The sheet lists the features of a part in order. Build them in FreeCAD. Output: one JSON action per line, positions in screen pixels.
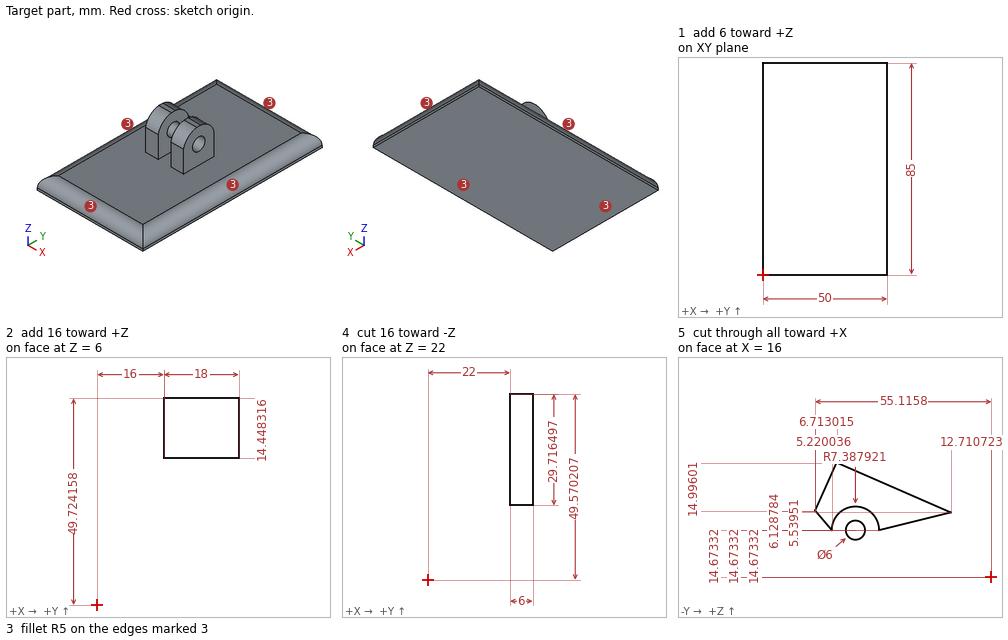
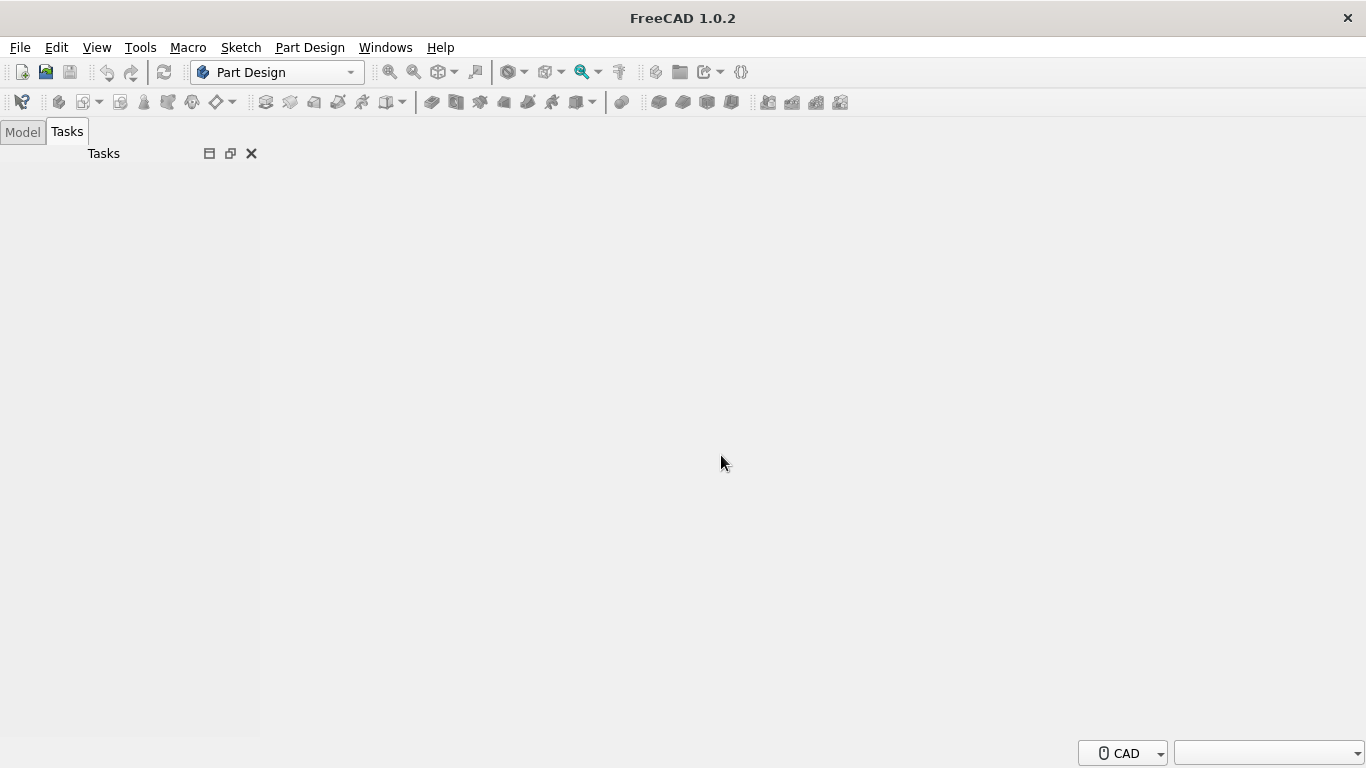
{"action": "key", "text": "ctrl+n"}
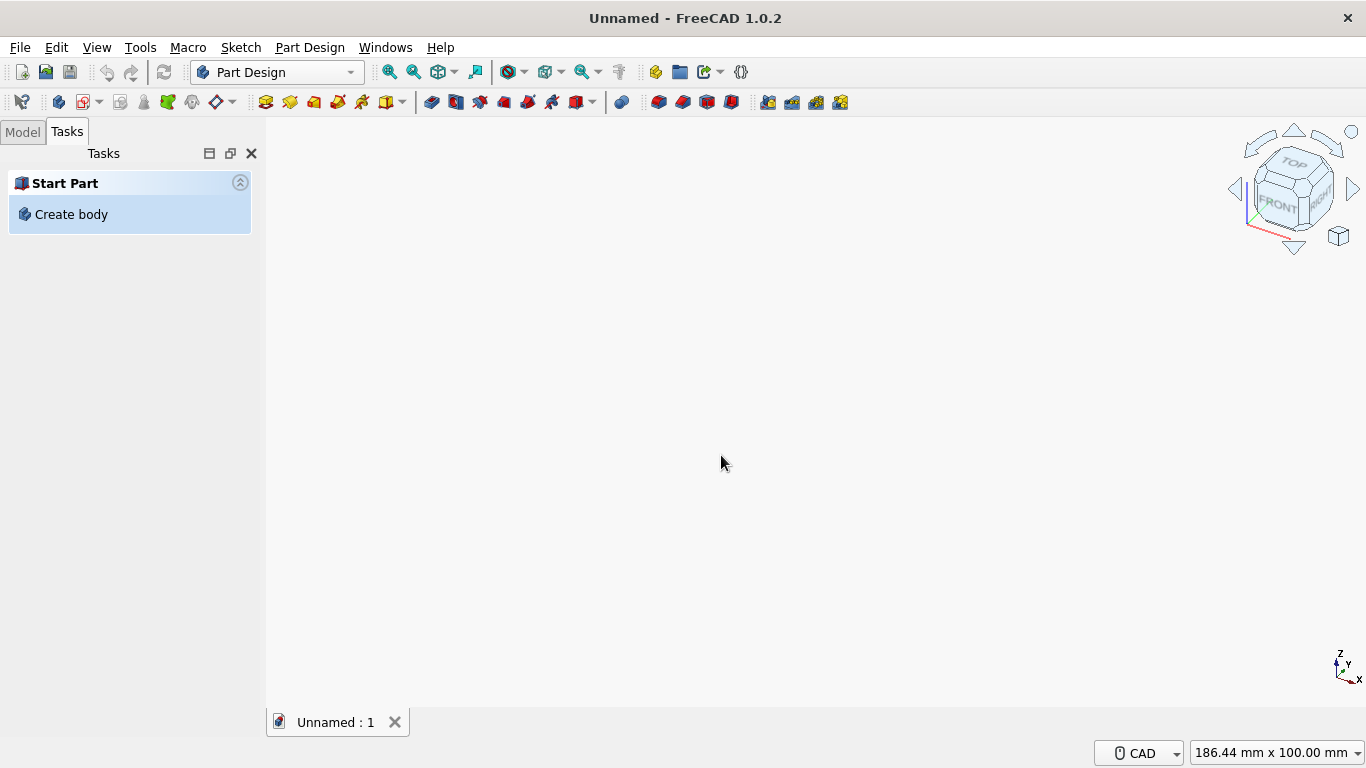
{"action": "left_click", "coordinate": [84, 102]}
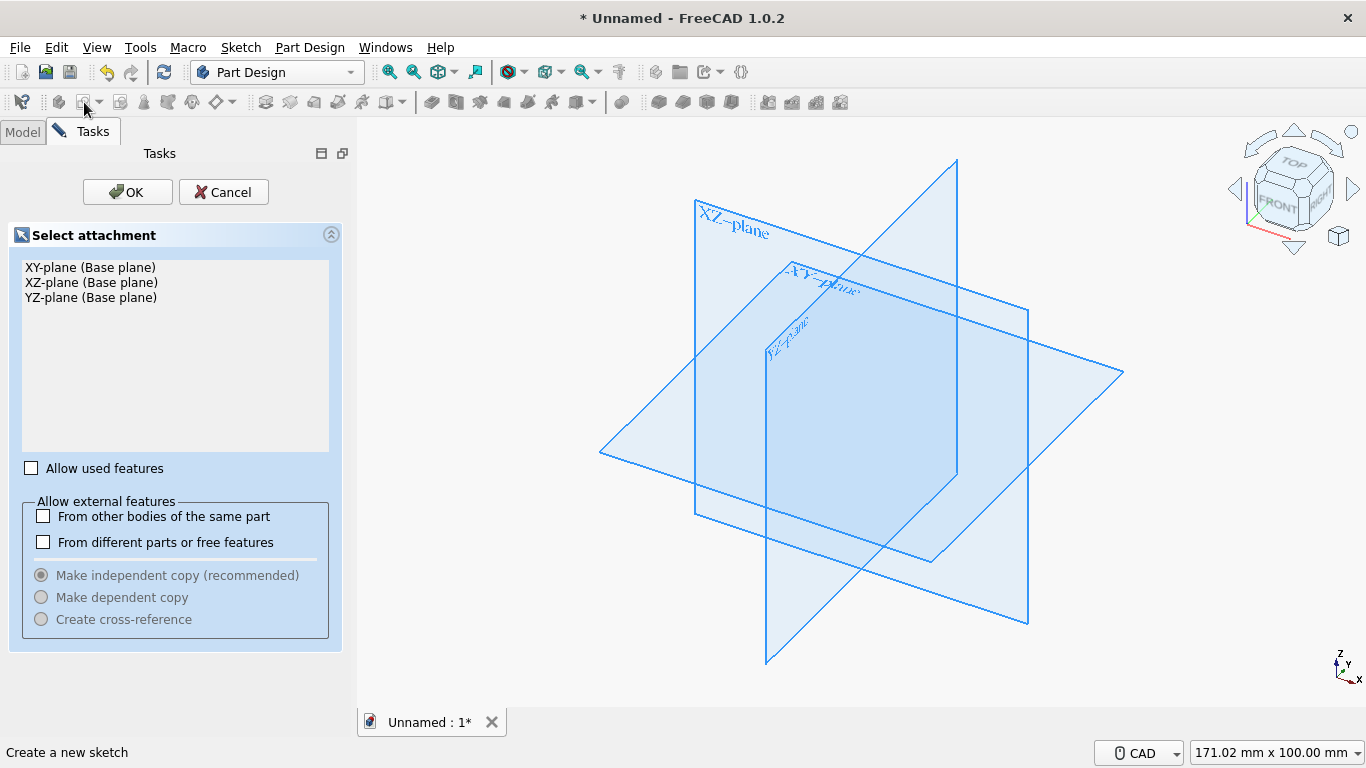
{"action": "left_click", "coordinate": [82, 268]}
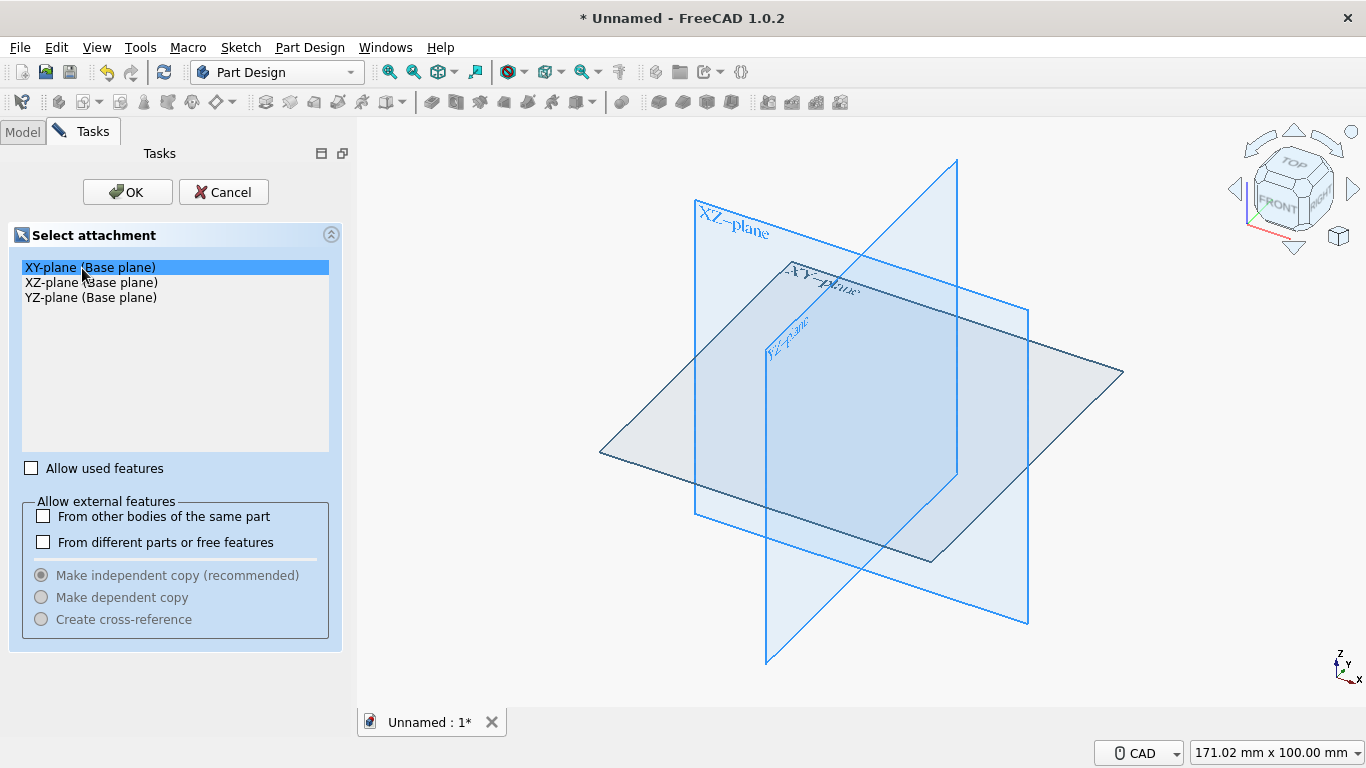
{"action": "left_click", "coordinate": [128, 192]}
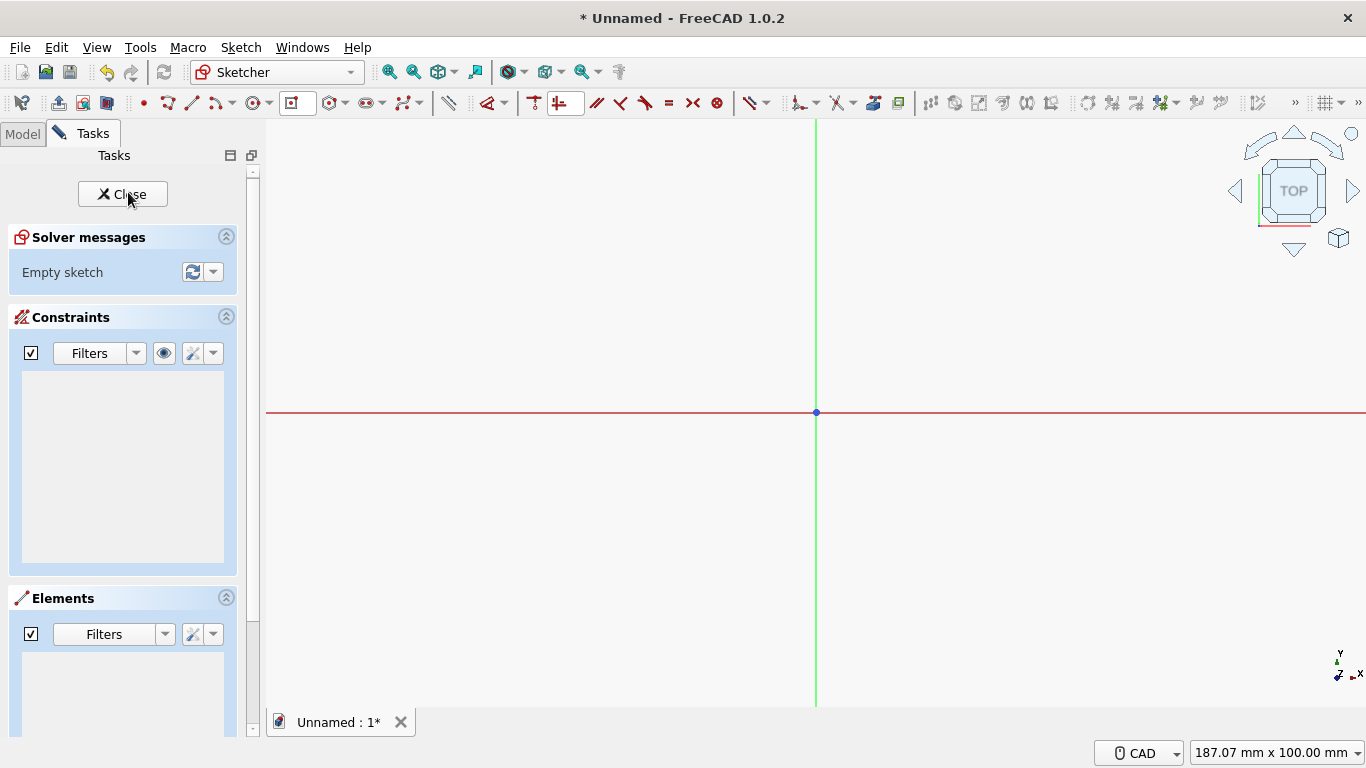
{"action": "scroll", "coordinate": [485, 679], "scroll_direction": "down", "scroll_amount": 3}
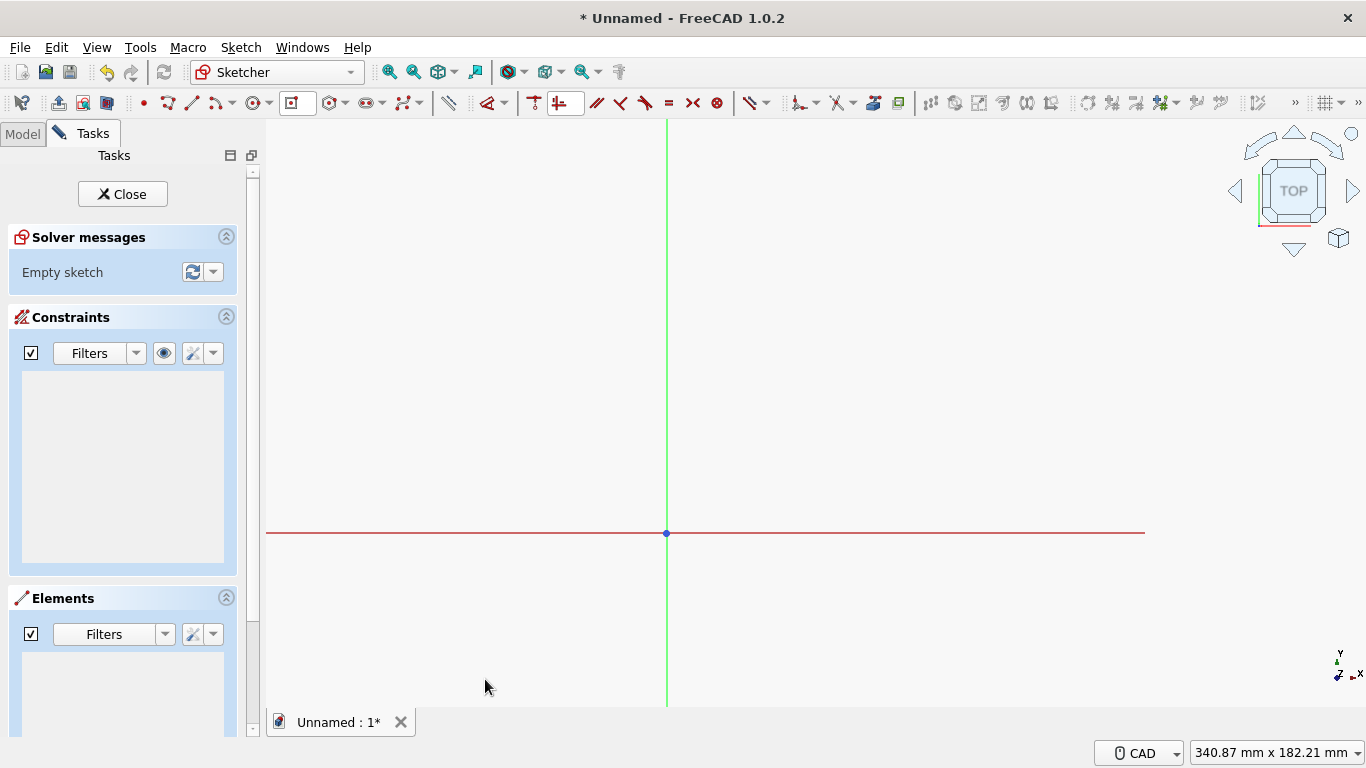
{"action": "scroll", "coordinate": [747, 362], "scroll_direction": "up", "scroll_amount": 2}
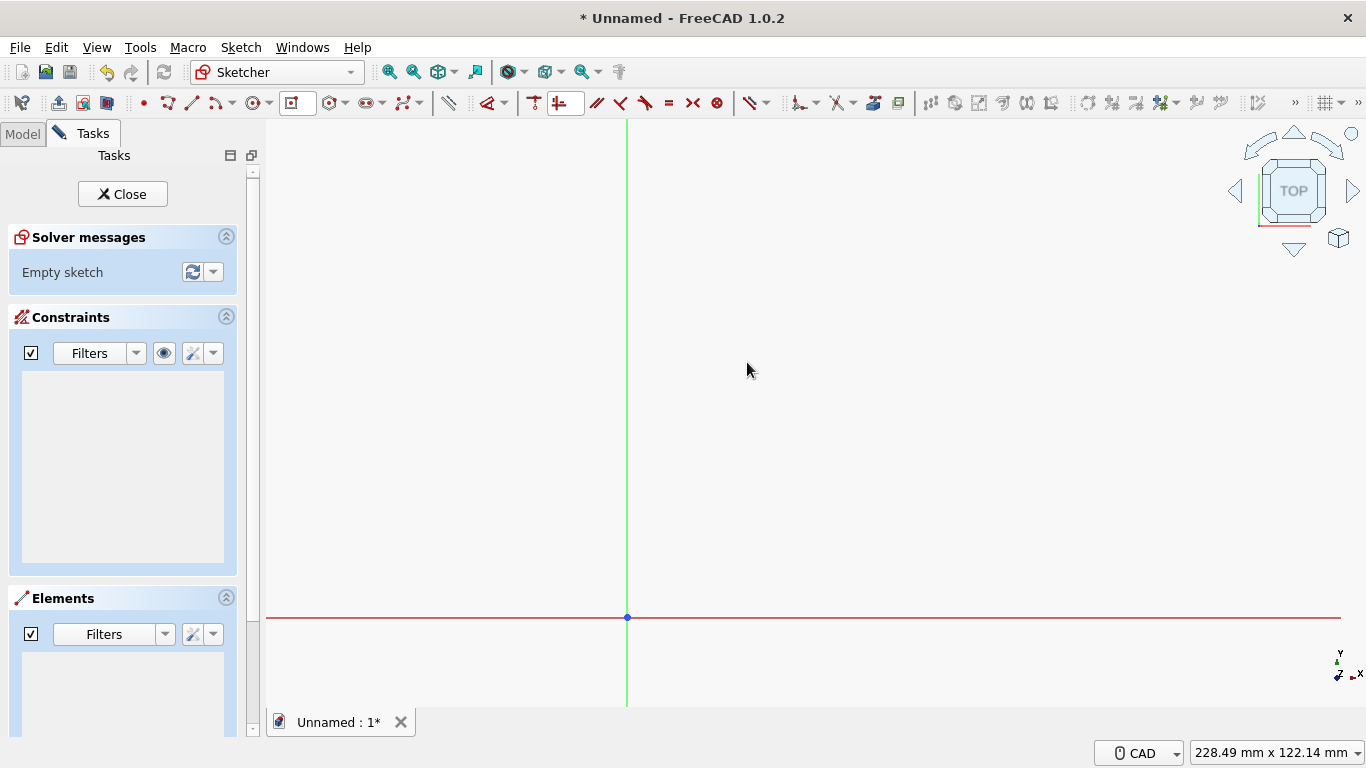
{"action": "key", "text": "g r"}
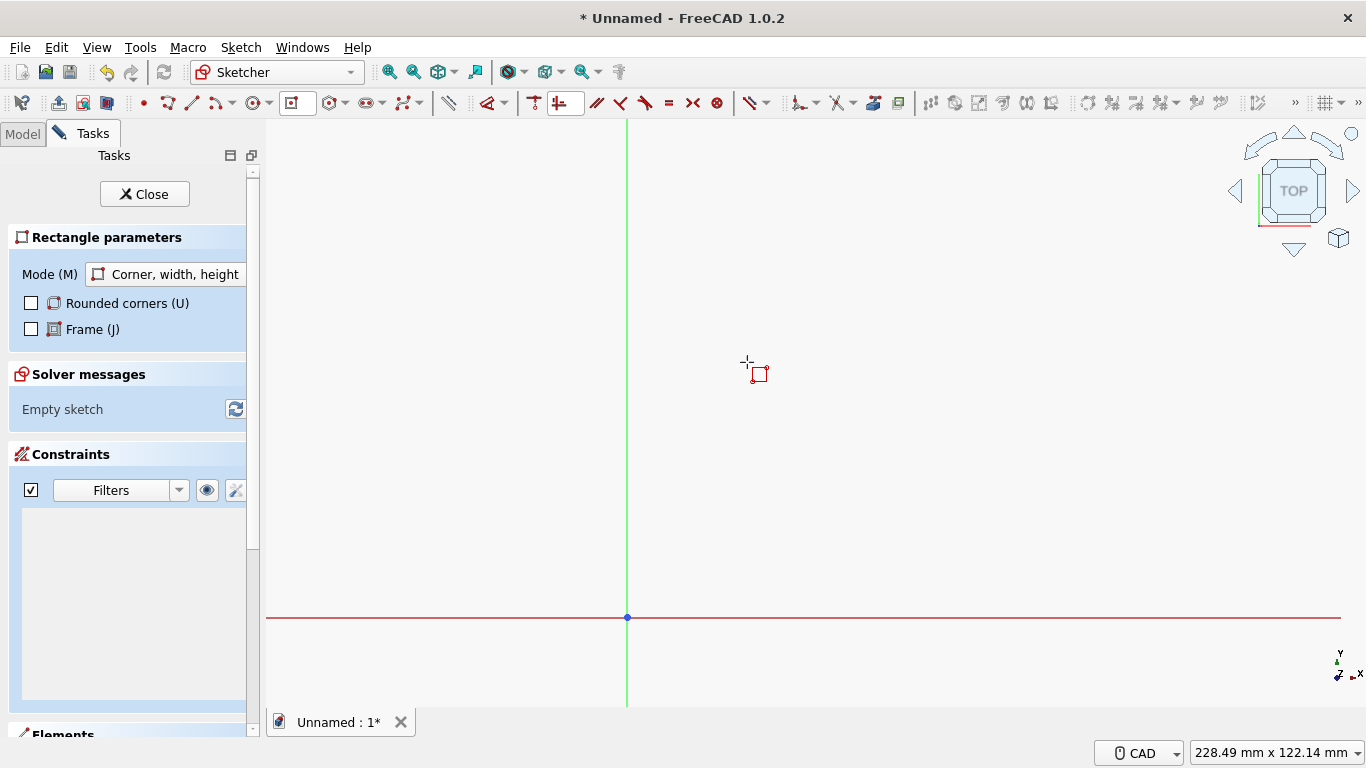
{"action": "left_click", "coordinate": [627, 618]}
{"action": "mouse_move", "coordinate": [868, 208]}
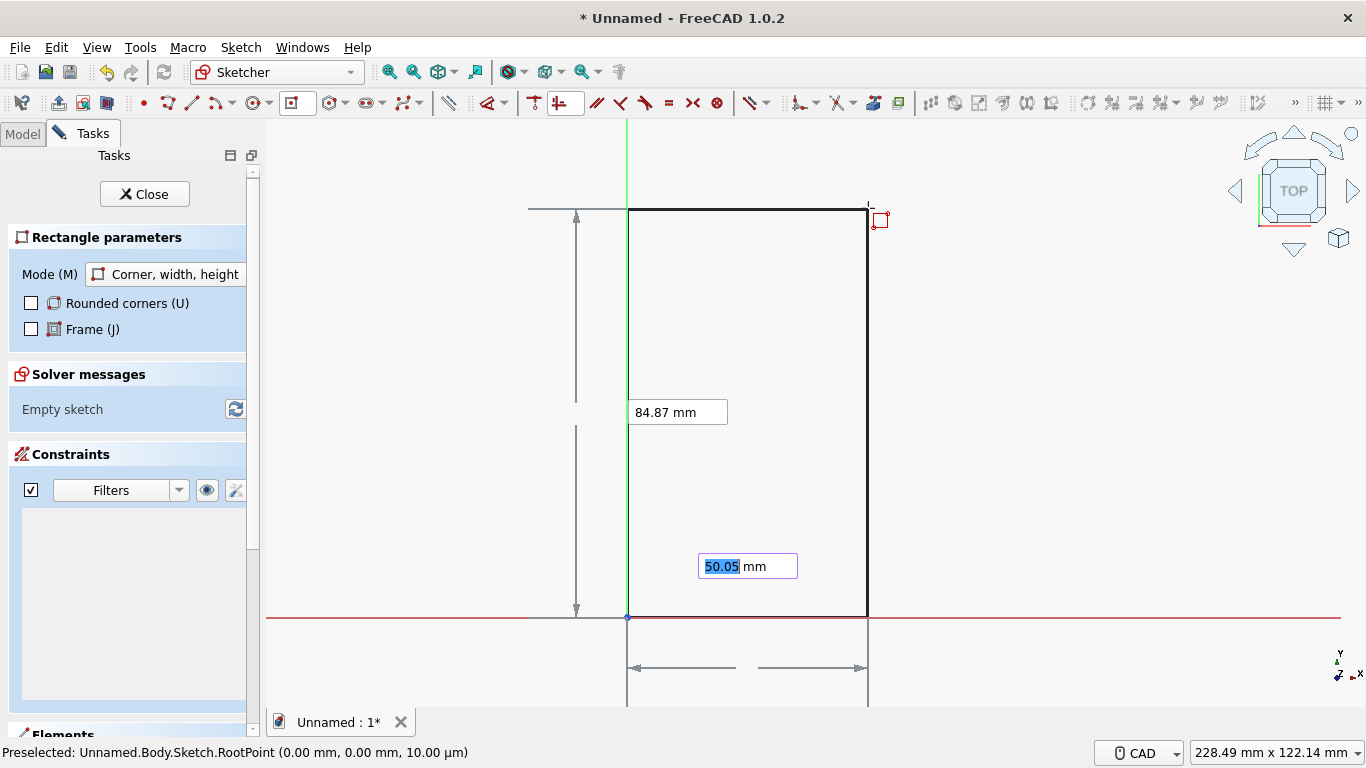
{"action": "type", "text": "50"}
{"action": "key", "text": "Tab"}
{"action": "type", "text": "85"}
{"action": "key", "text": "Return"}
{"action": "key", "text": "Escape"}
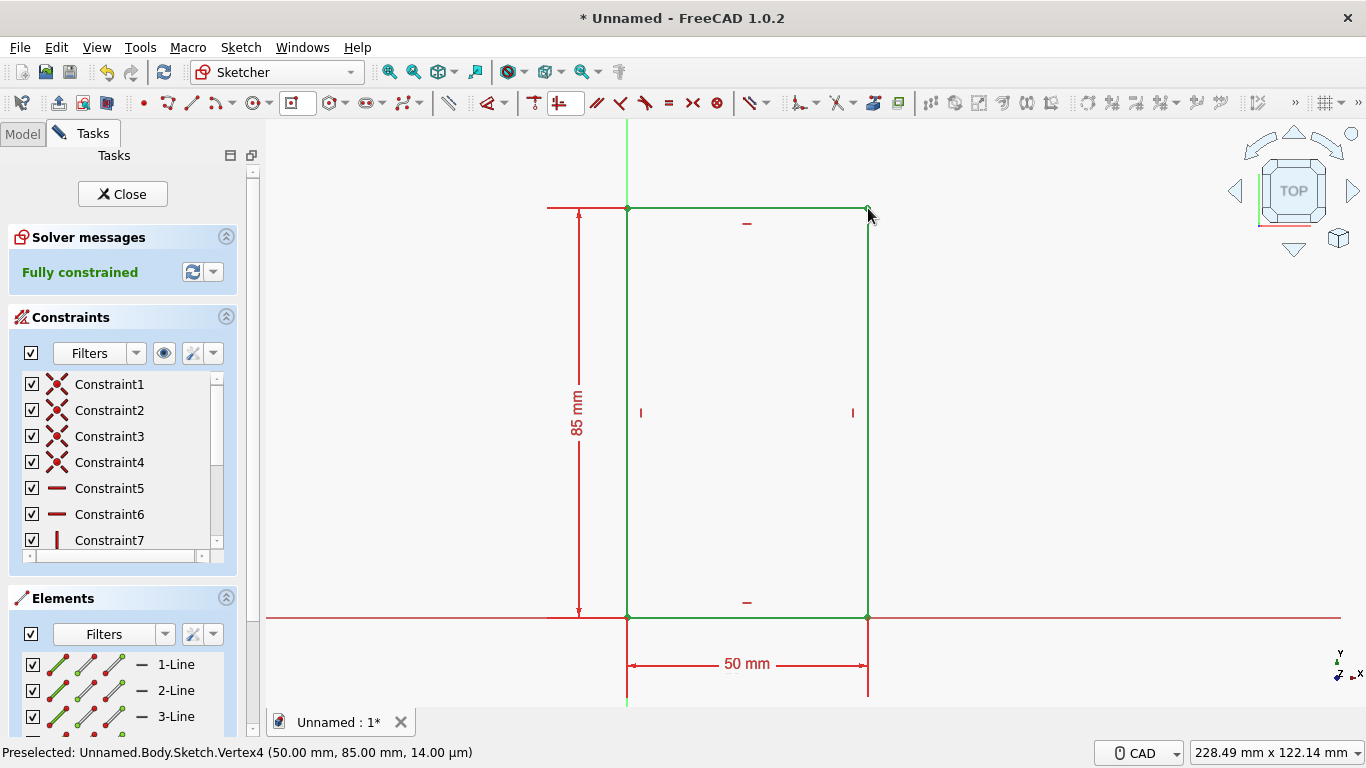
{"action": "left_click", "coordinate": [123, 194]}